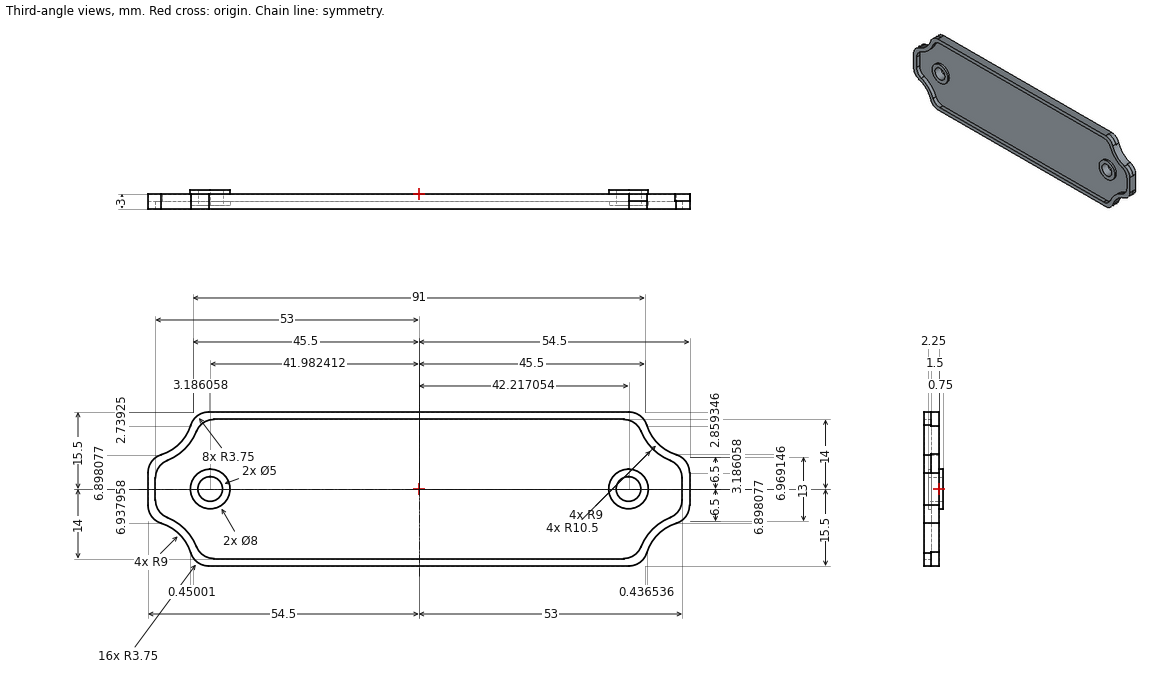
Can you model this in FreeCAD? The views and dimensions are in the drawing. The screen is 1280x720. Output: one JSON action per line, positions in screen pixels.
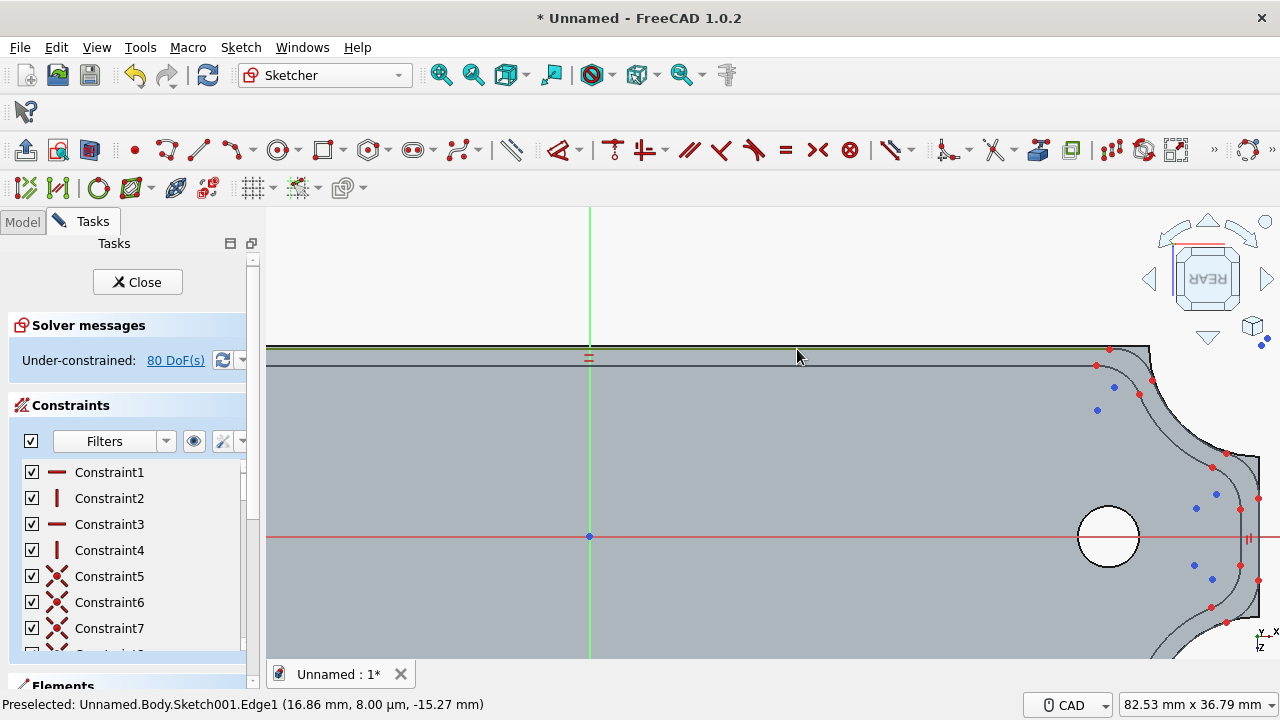
{"action": "scroll", "coordinate": [798, 348], "scroll_direction": "down", "scroll_amount": 4}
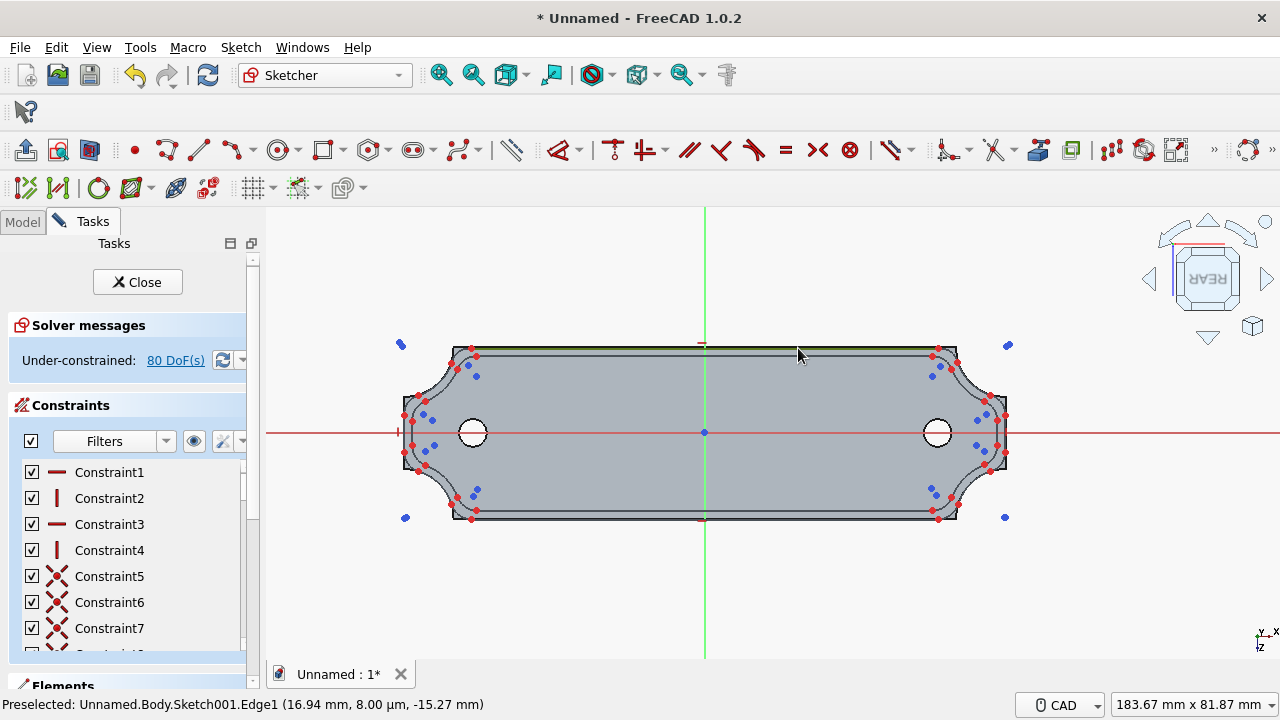
{"action": "scroll", "coordinate": [463, 349], "scroll_direction": "up", "scroll_amount": 3}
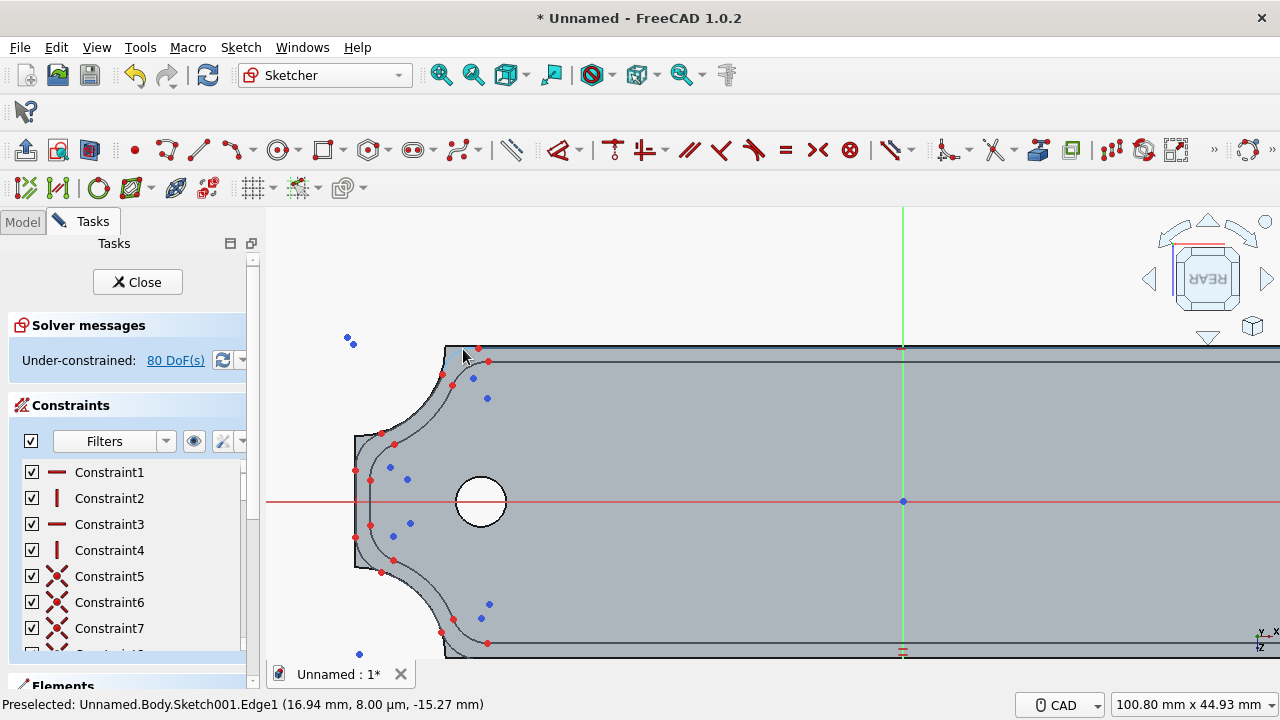
{"action": "left_click", "coordinate": [464, 349]}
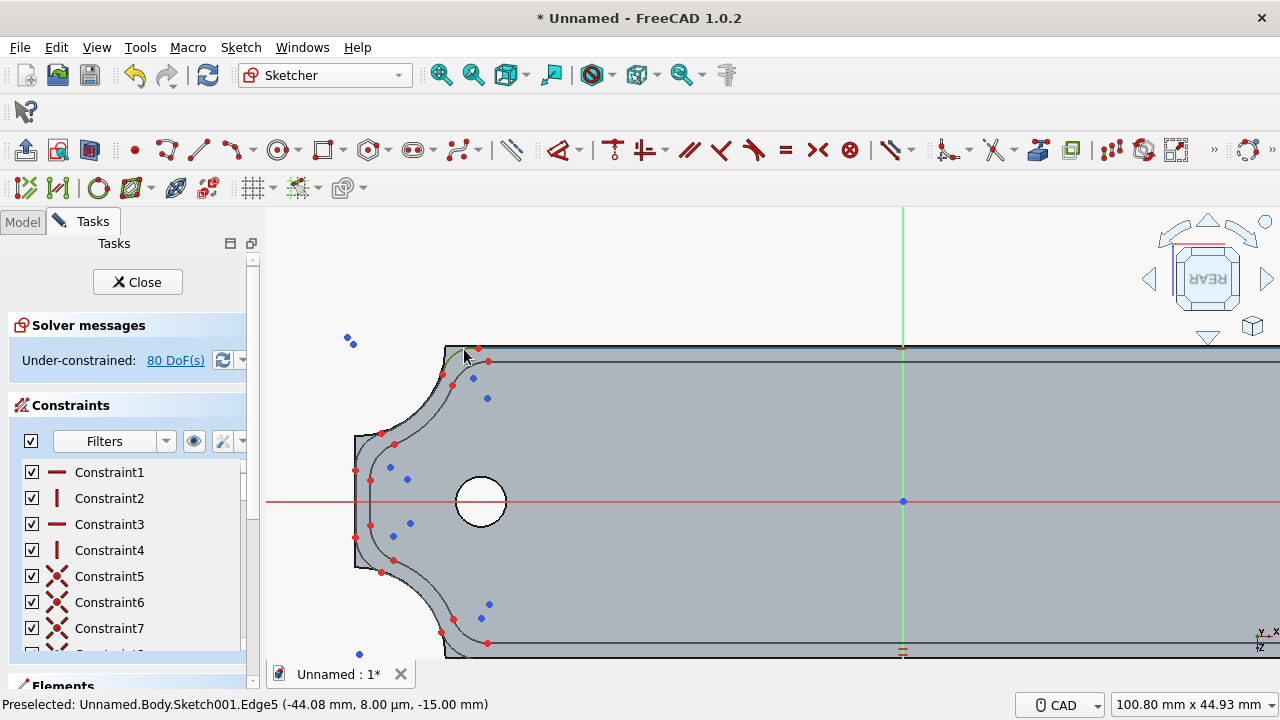
{"action": "left_click", "coordinate": [754, 150]}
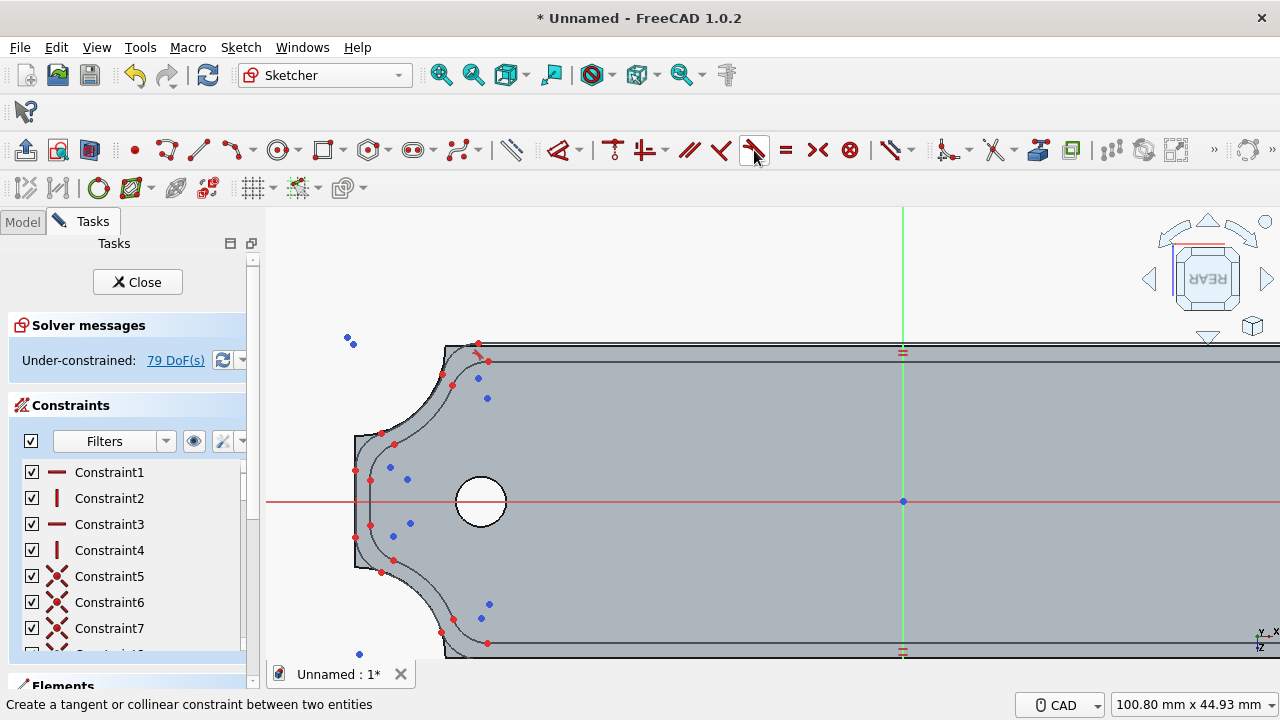
{"action": "left_click", "coordinate": [1073, 343]}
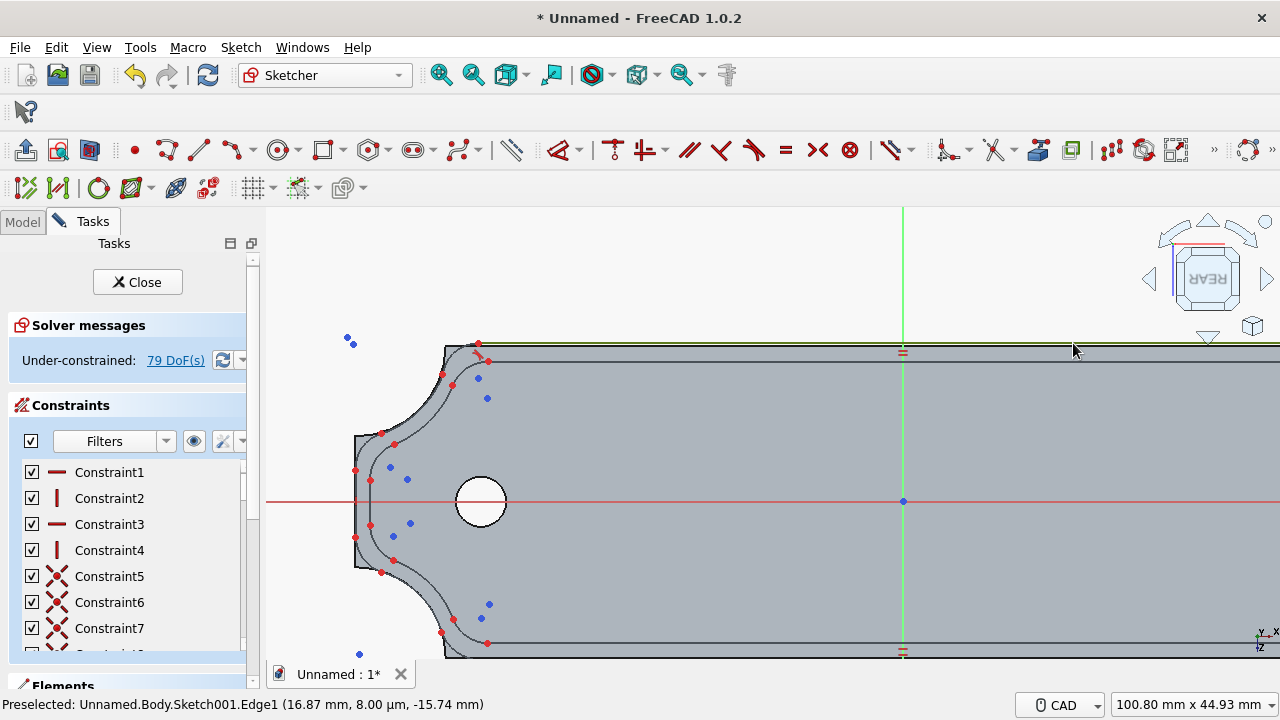
{"action": "scroll", "coordinate": [463, 349], "scroll_direction": "down", "scroll_amount": 3}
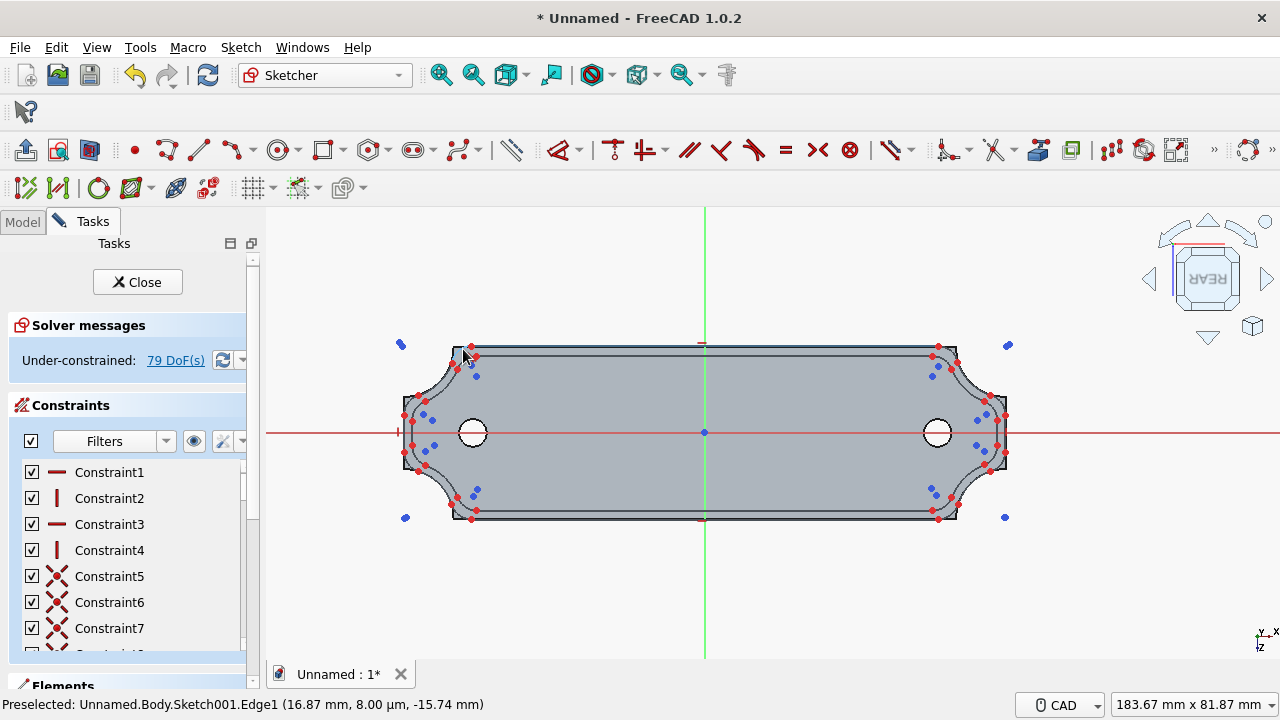
{"action": "scroll", "coordinate": [955, 355], "scroll_direction": "up", "scroll_amount": 3}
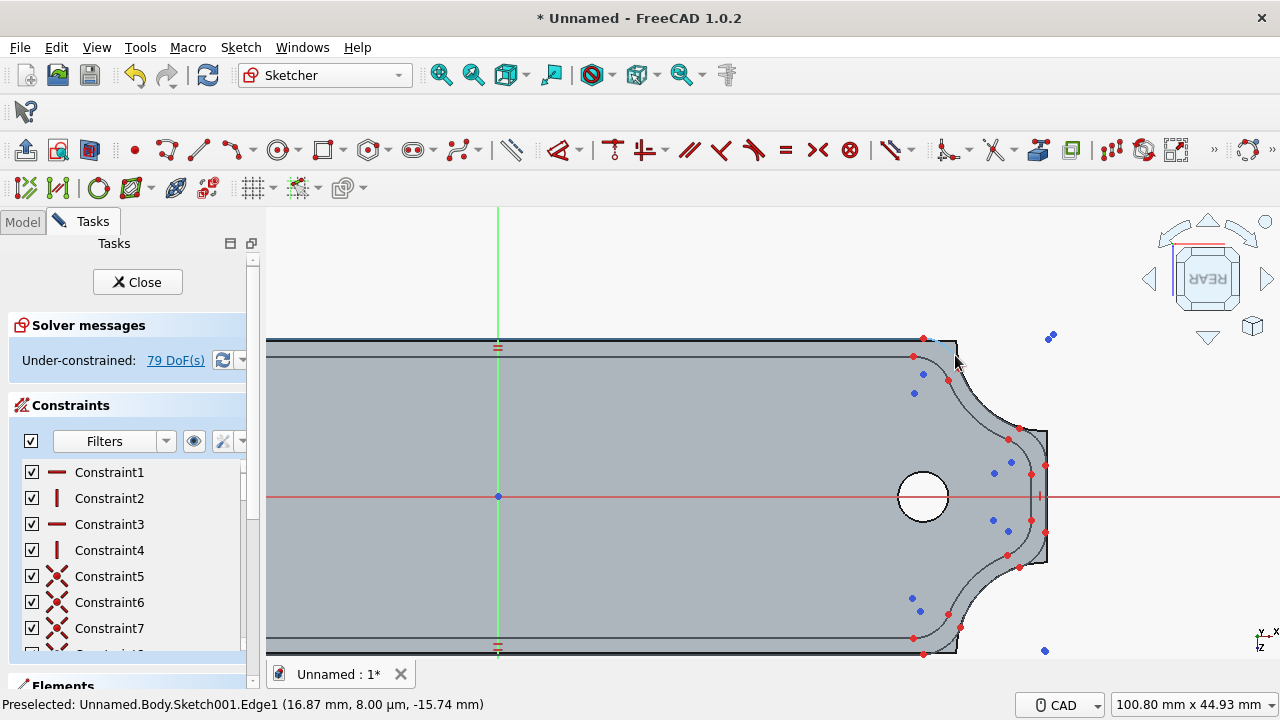
{"action": "left_click", "coordinate": [954, 355]}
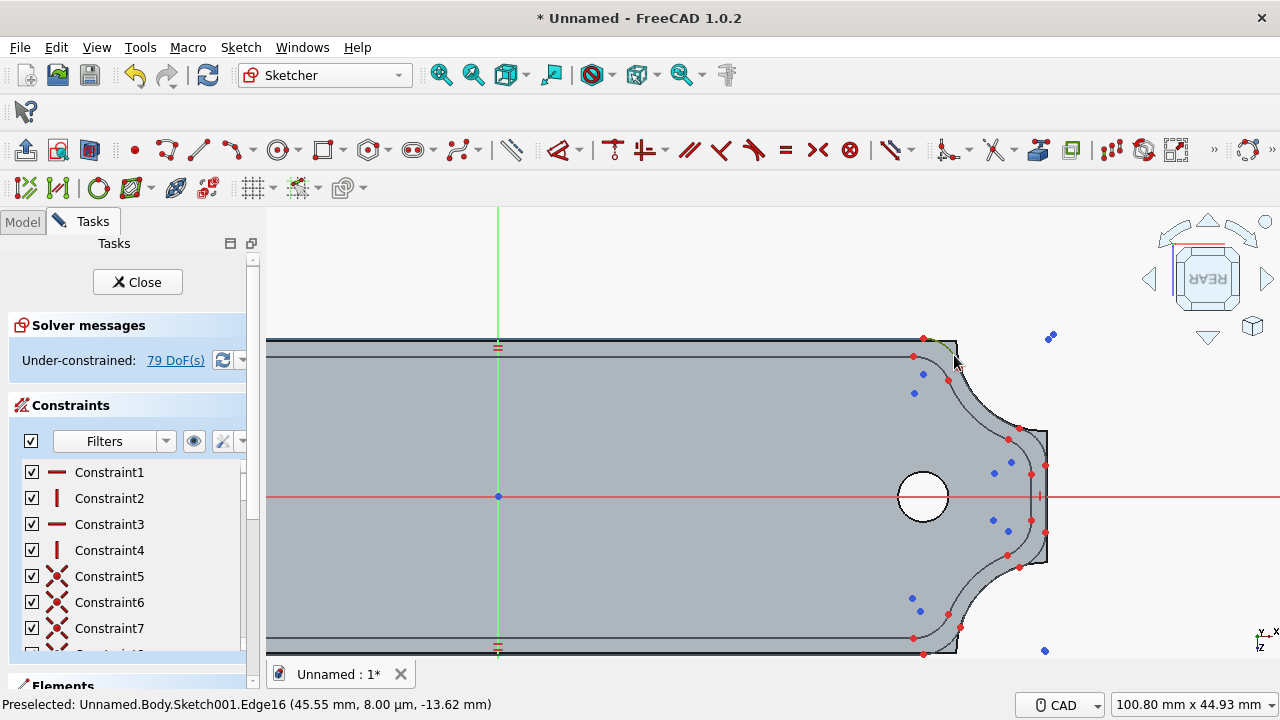
{"action": "left_click", "coordinate": [754, 150]}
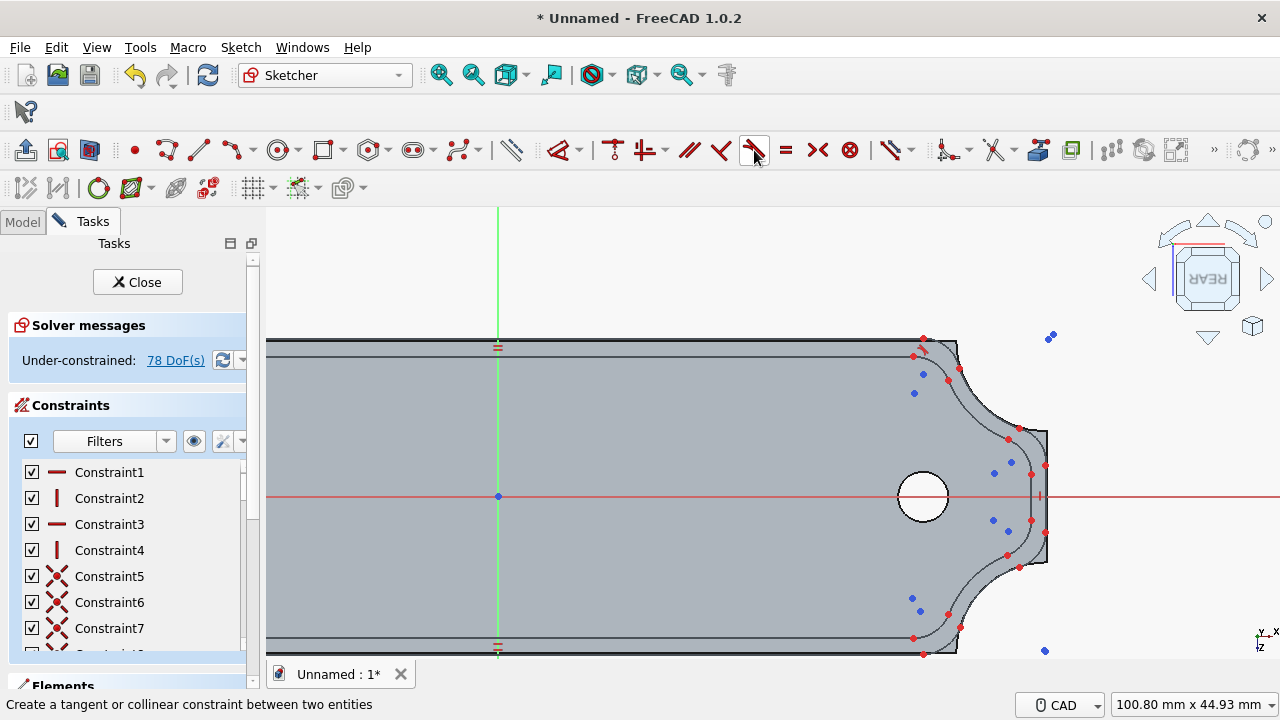
{"action": "scroll", "coordinate": [955, 355], "scroll_direction": "down", "scroll_amount": 3}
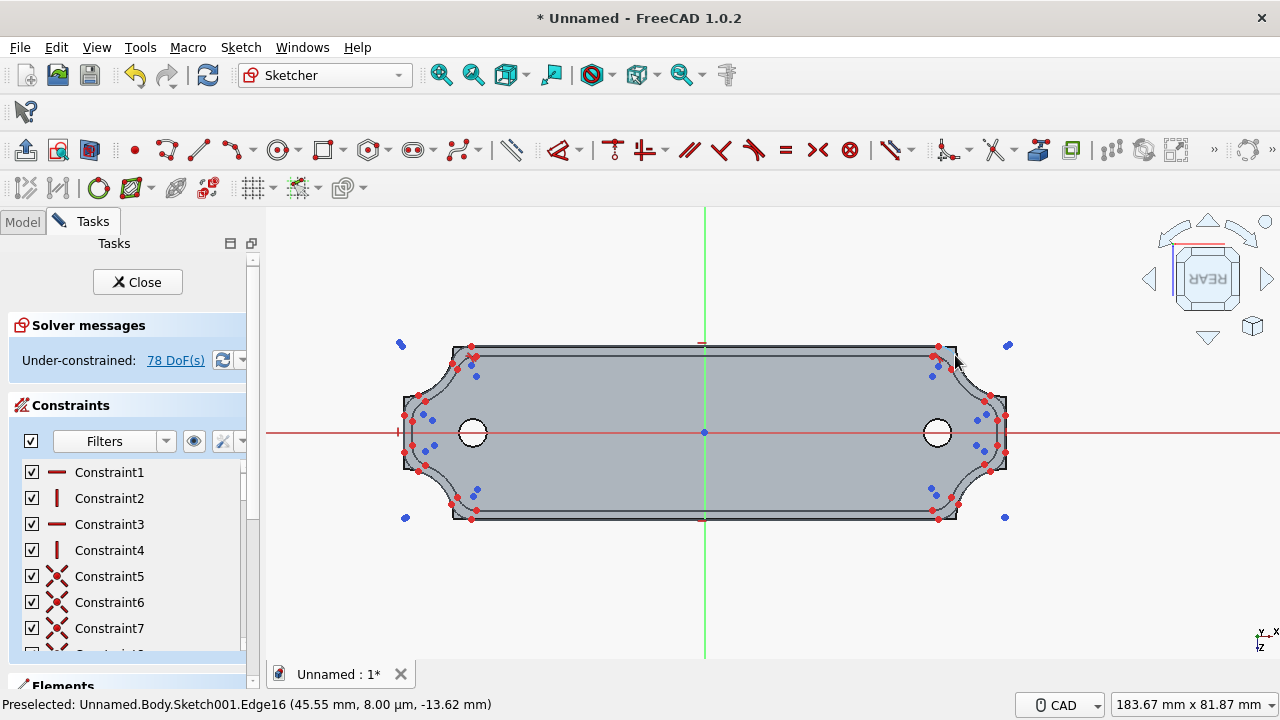
{"action": "scroll", "coordinate": [404, 427], "scroll_direction": "up", "scroll_amount": 5}